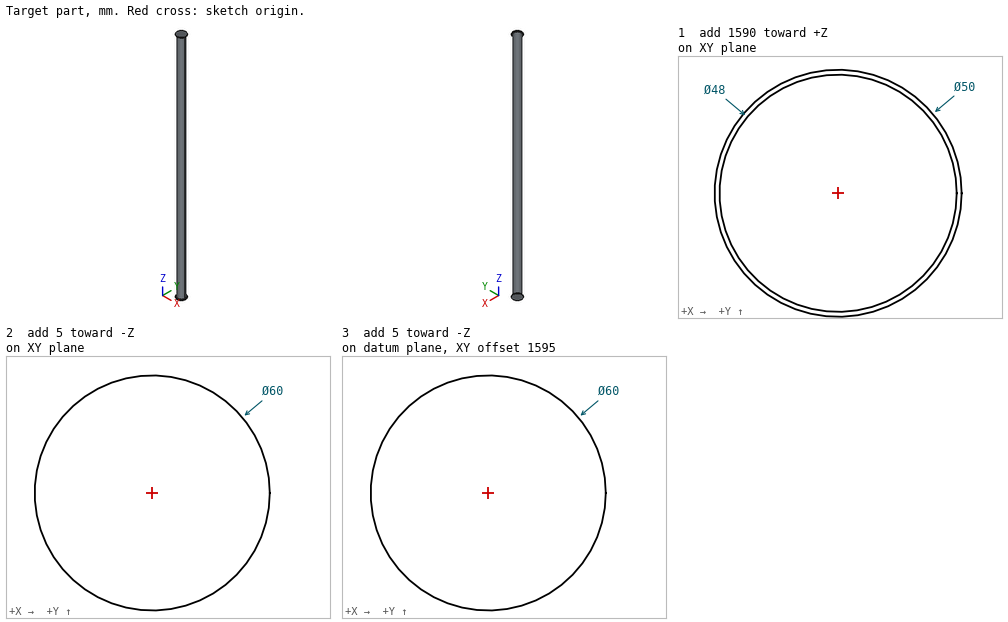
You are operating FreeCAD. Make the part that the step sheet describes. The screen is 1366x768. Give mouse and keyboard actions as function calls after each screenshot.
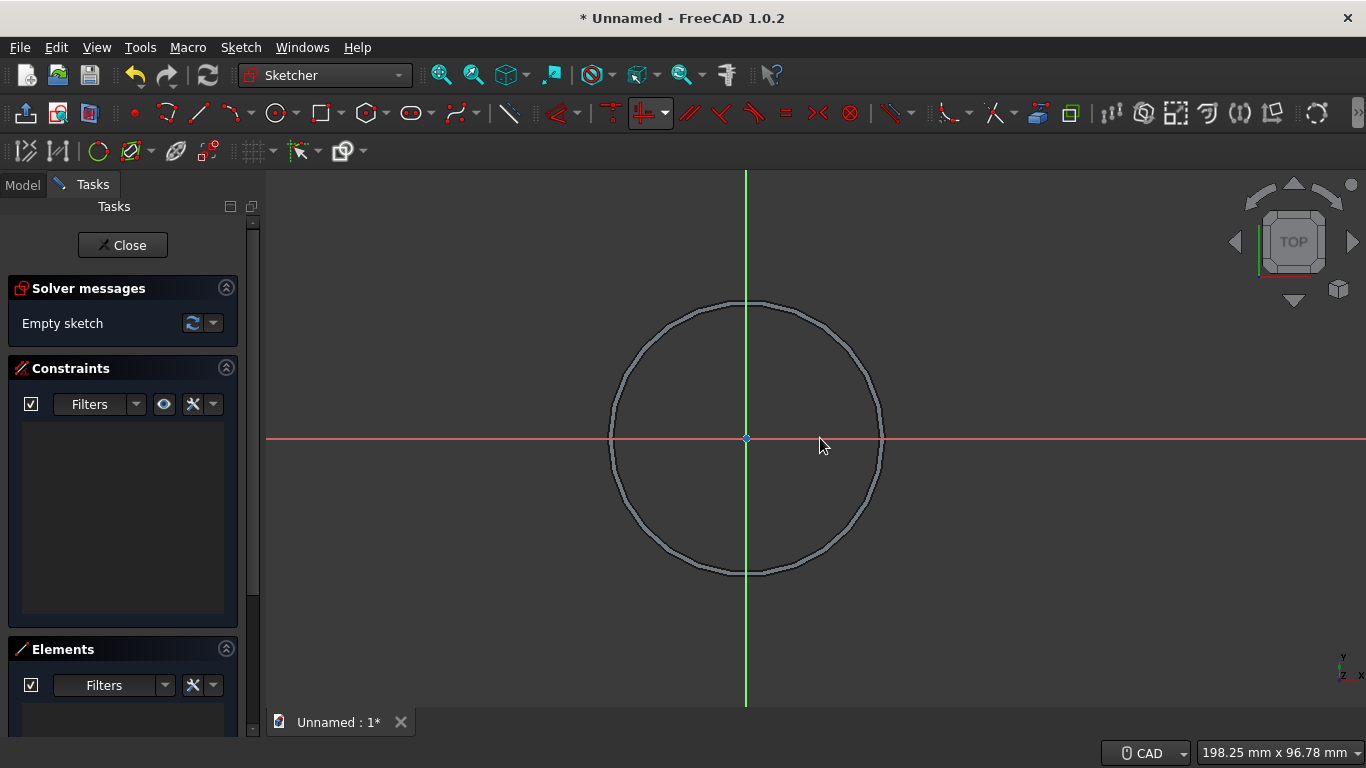
click(276, 114)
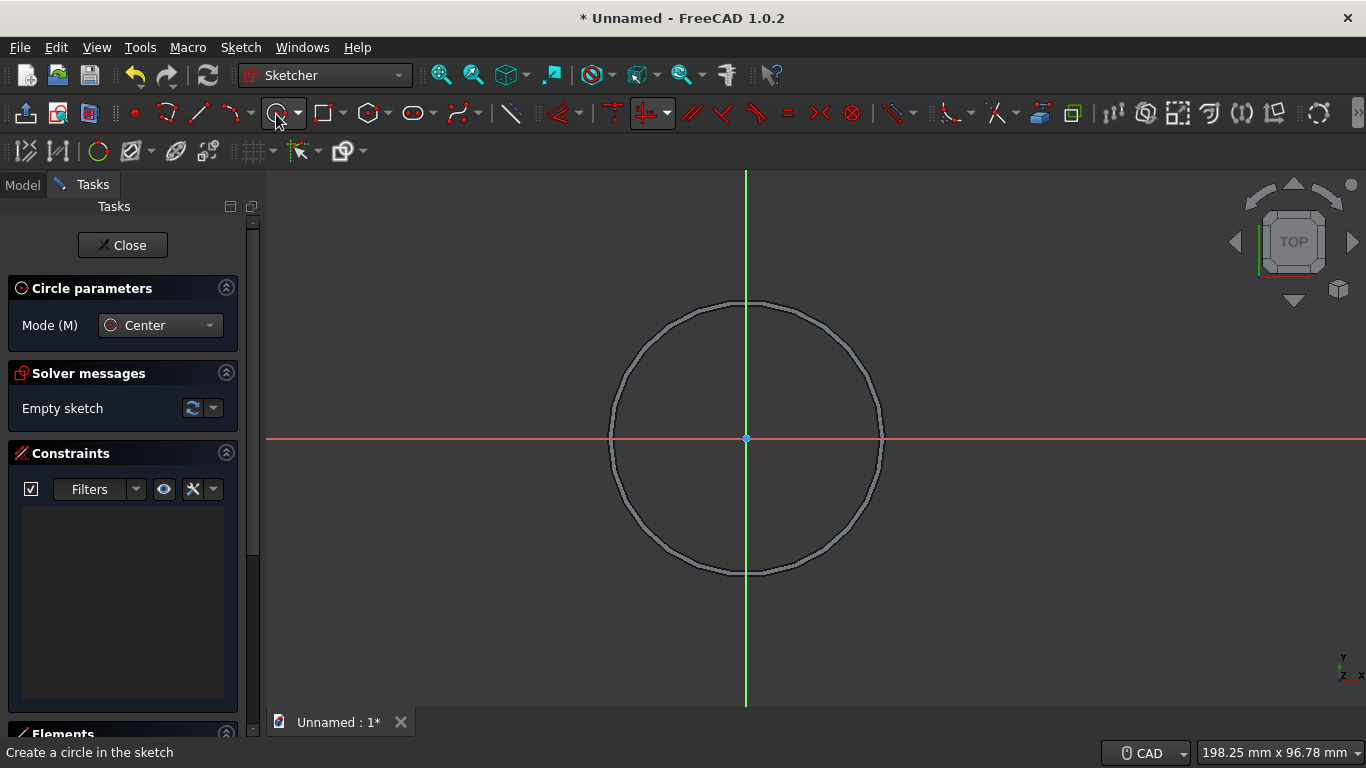
click(746, 438)
move(864, 321)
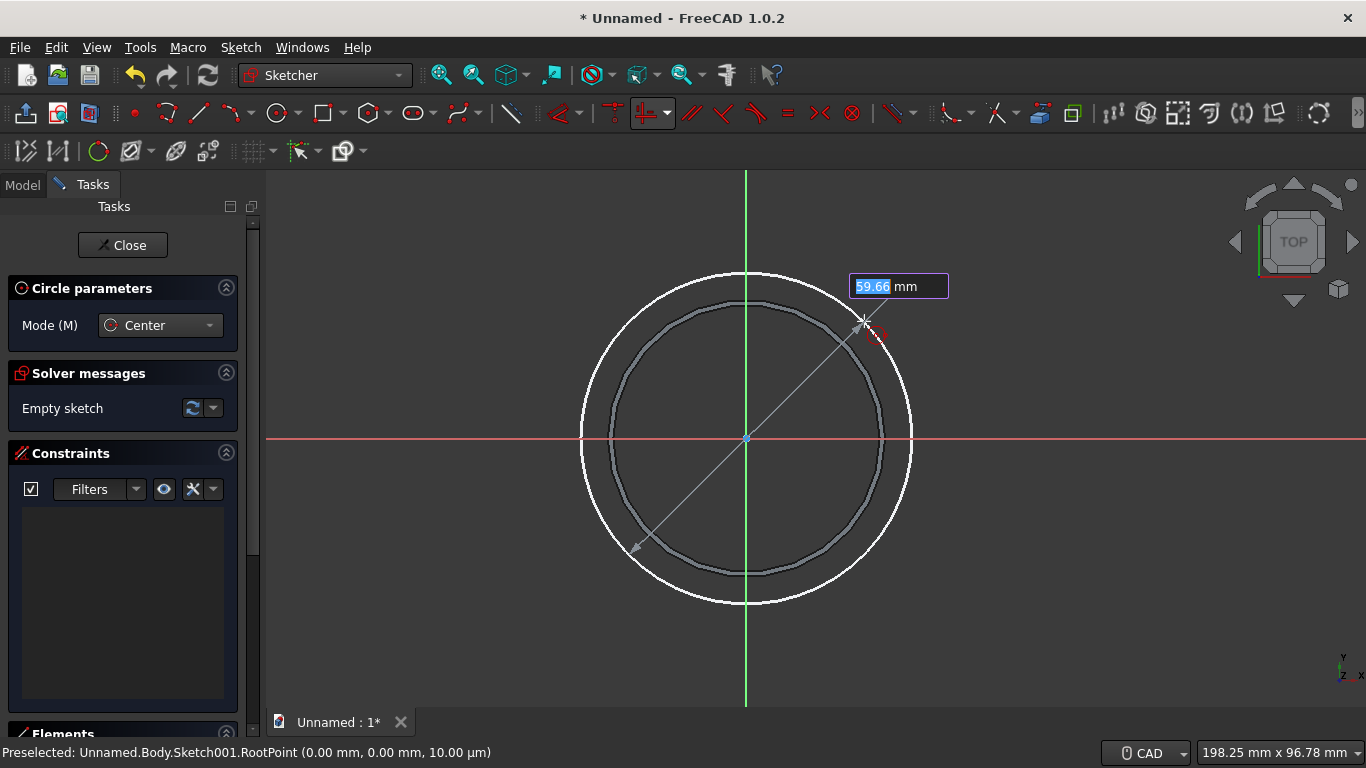
text(60)
key(Return)
key(Escape)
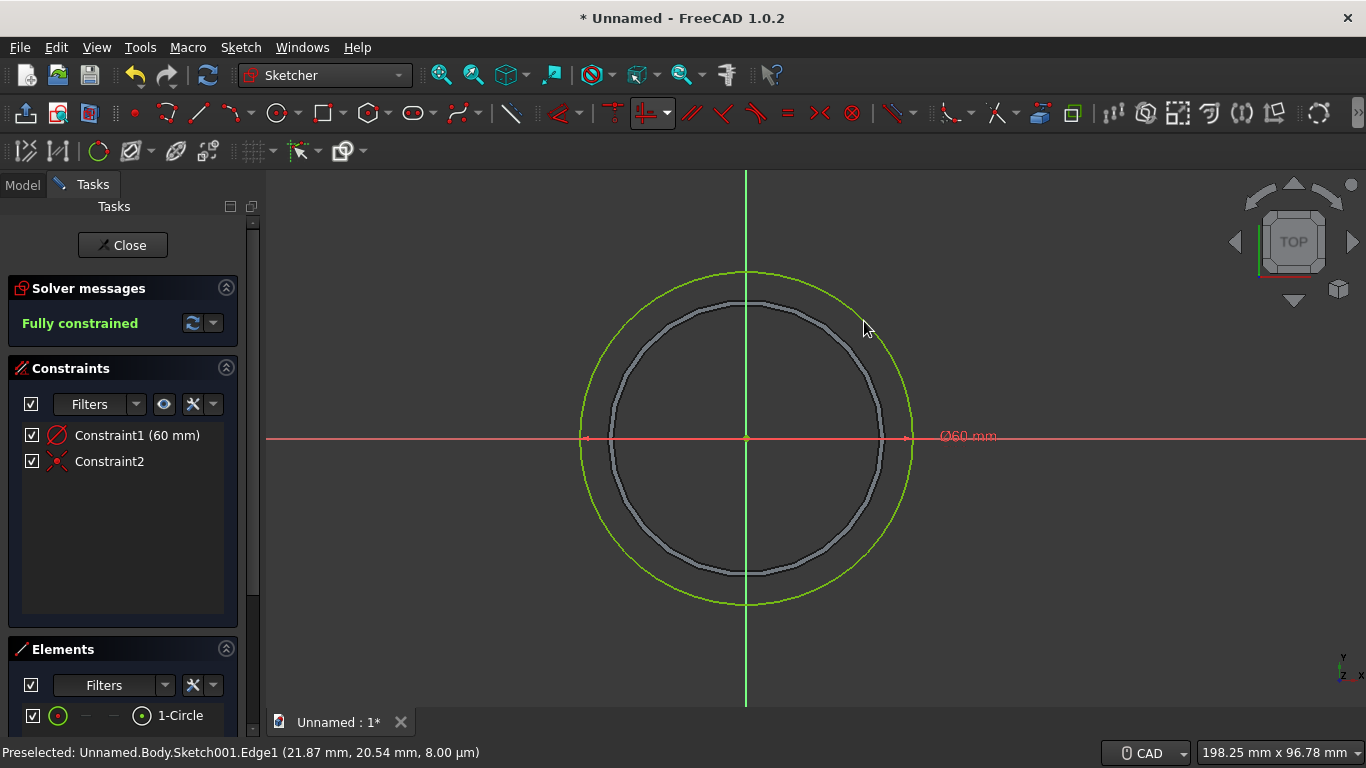
click(123, 245)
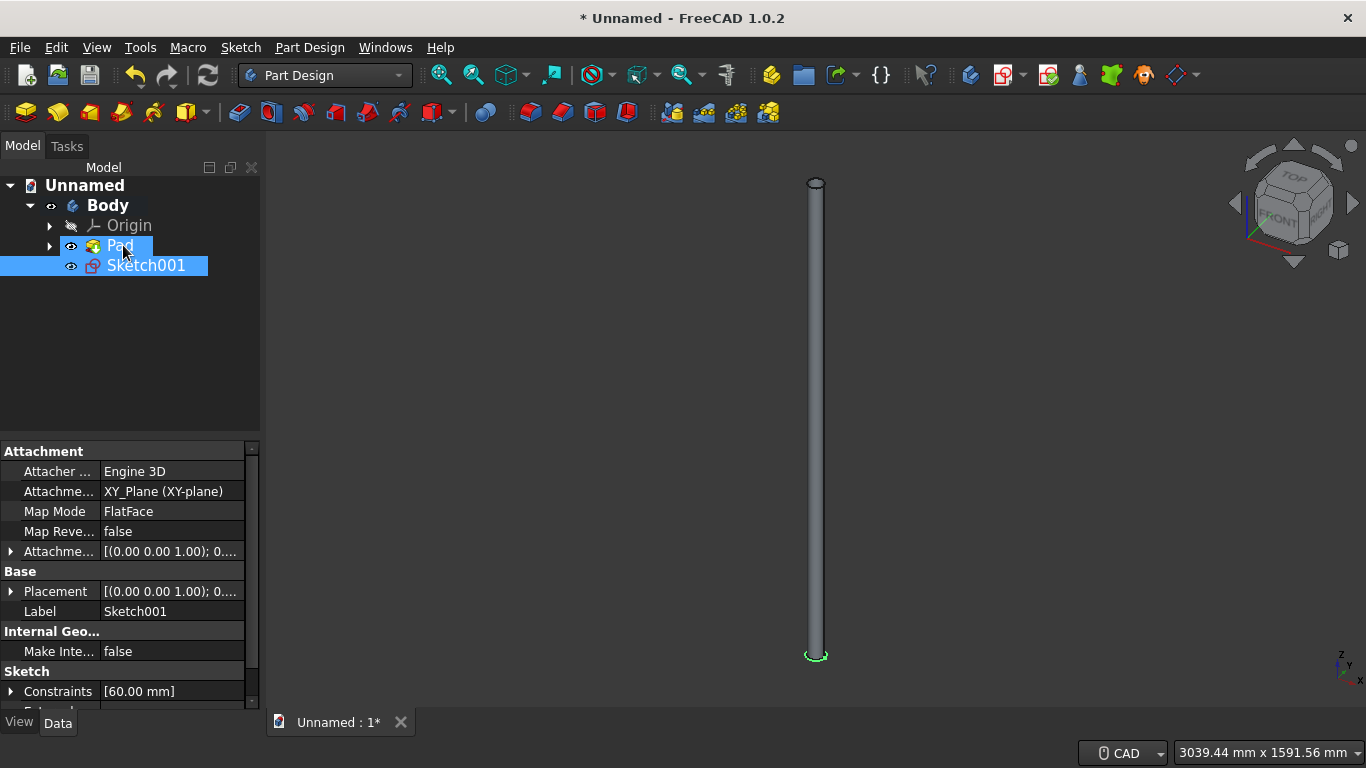
click(26, 112)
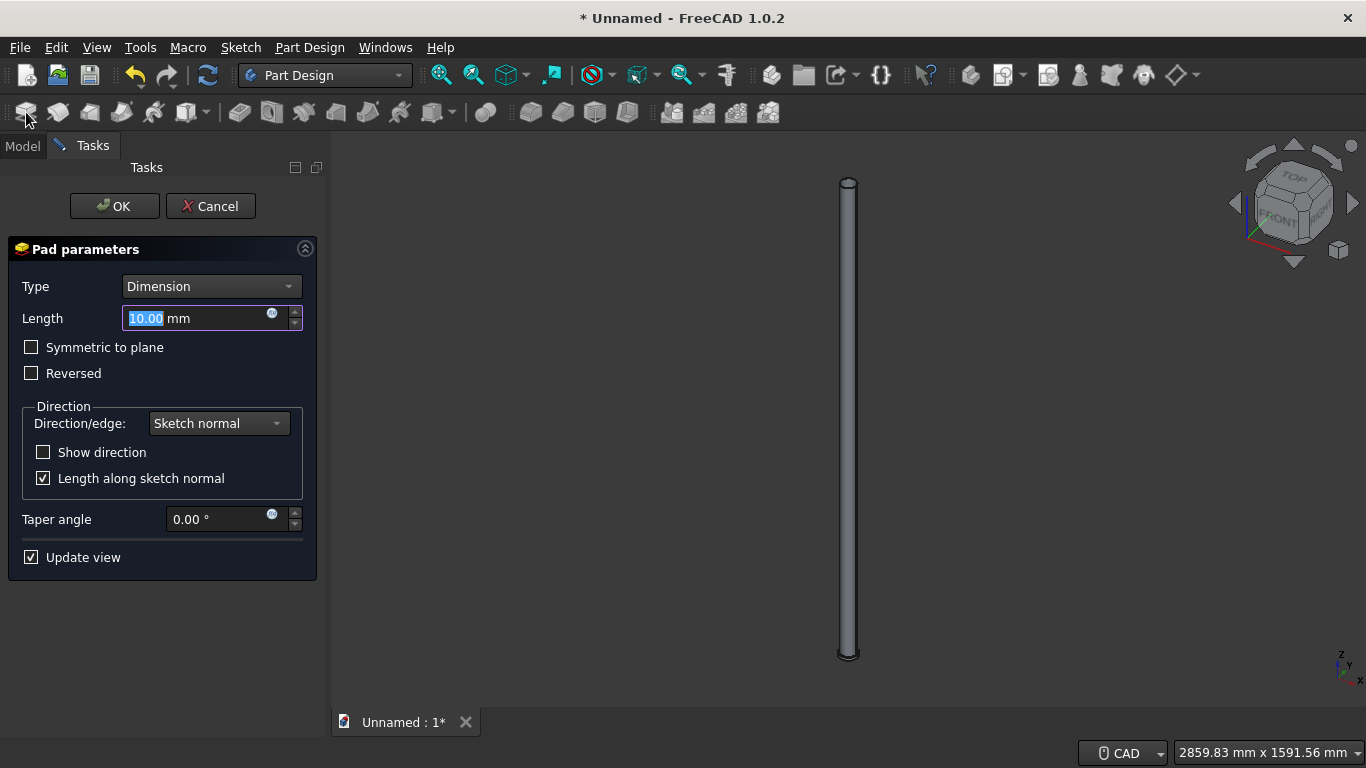
text(5)
key(Tab)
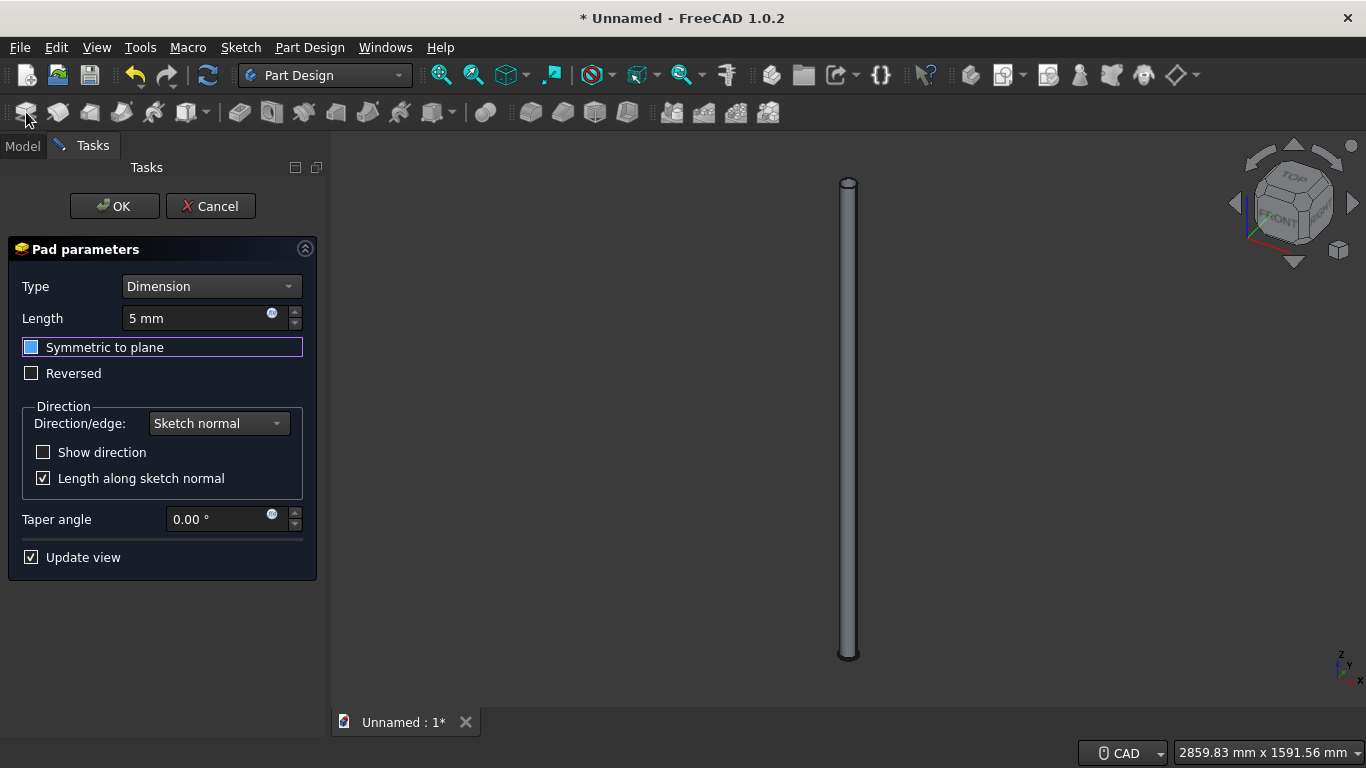
click(30, 373)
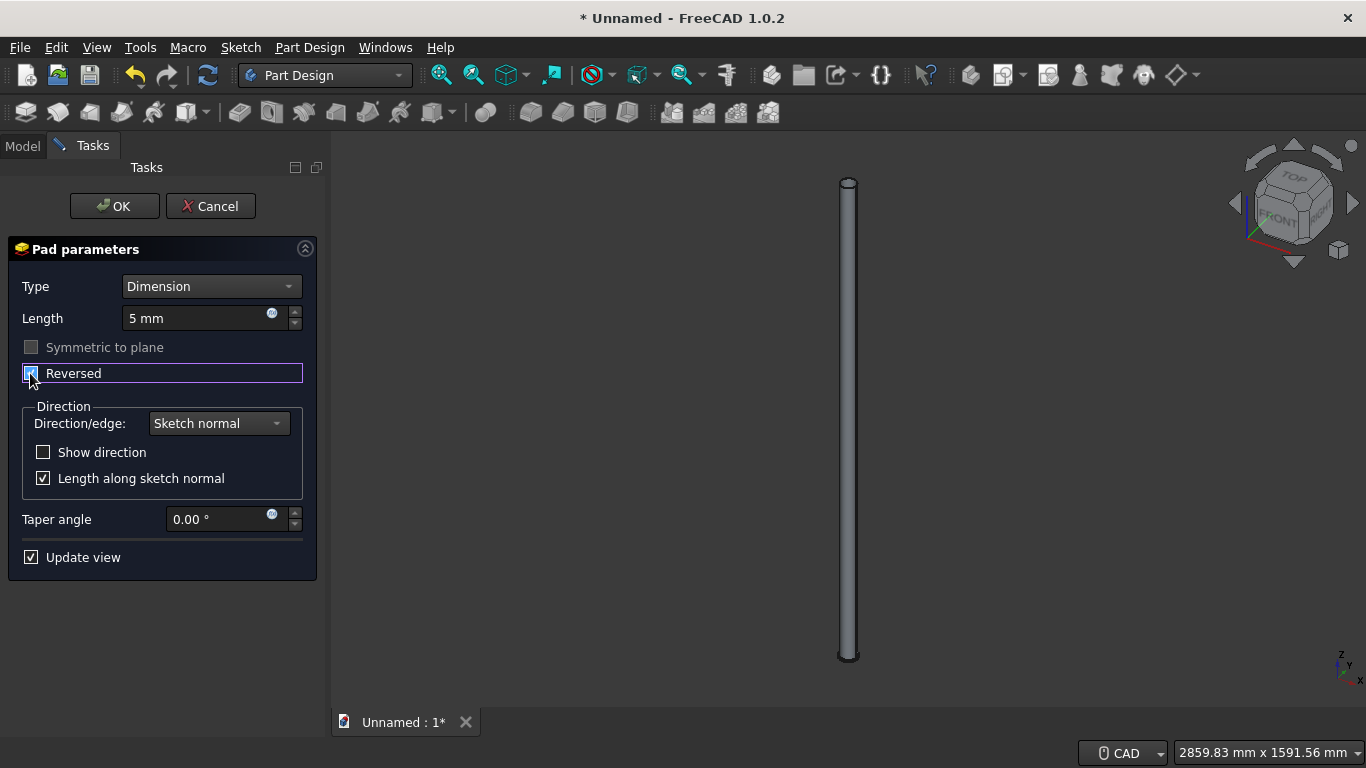
click(115, 206)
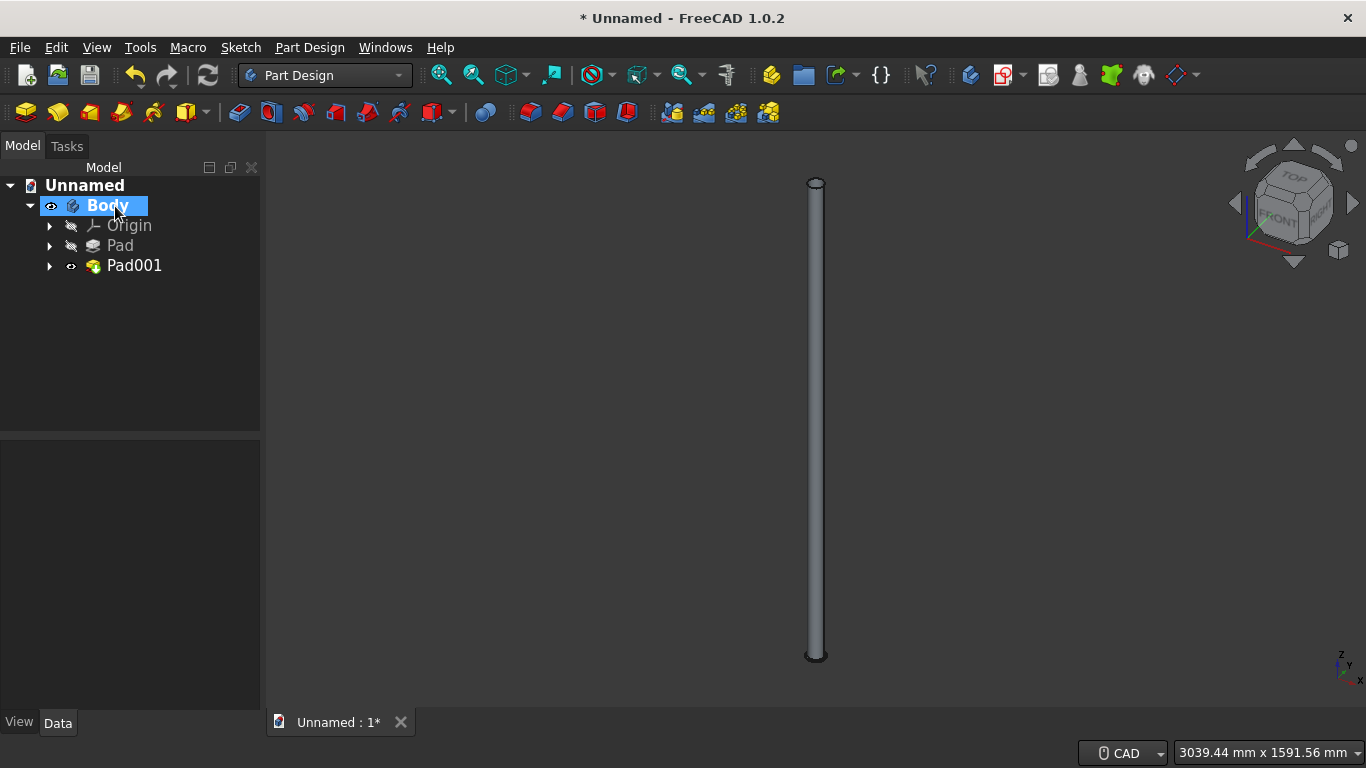
click(50, 226)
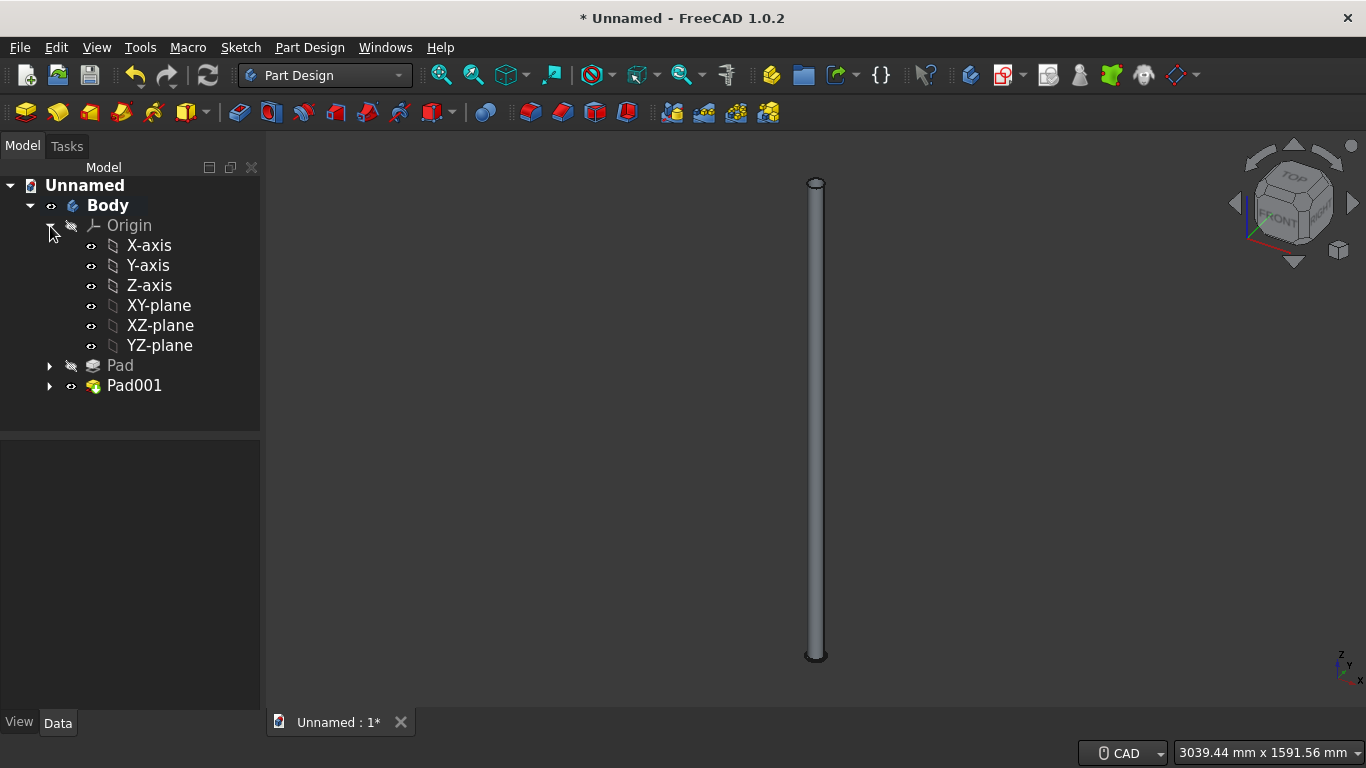
click(136, 306)